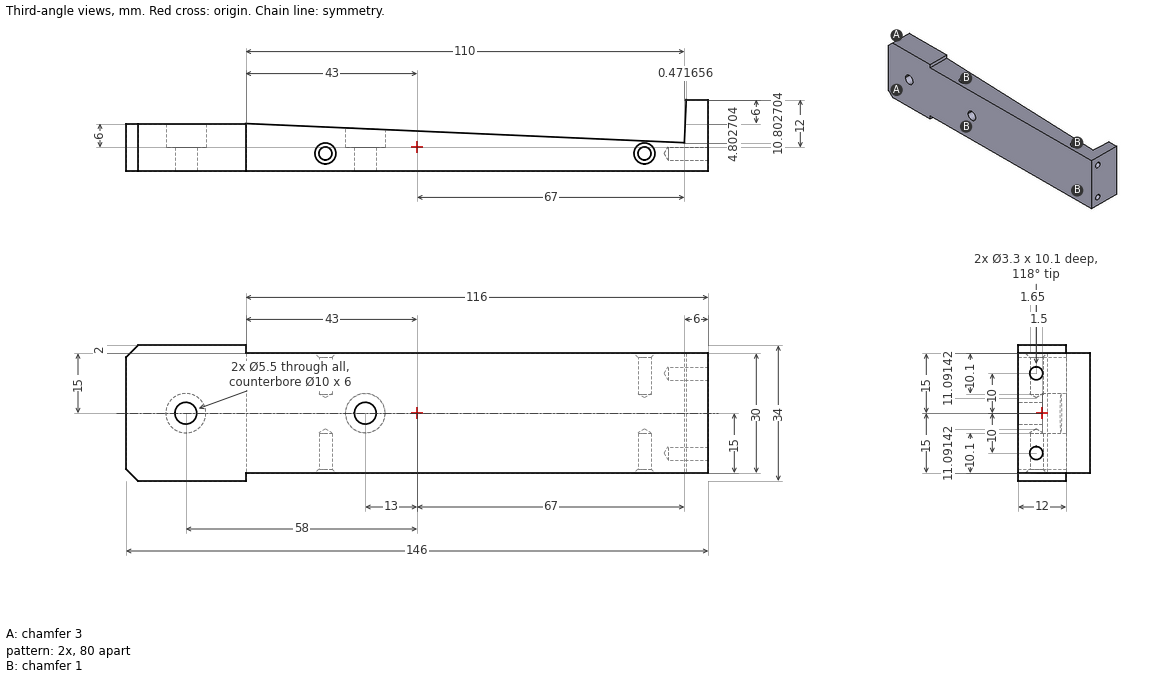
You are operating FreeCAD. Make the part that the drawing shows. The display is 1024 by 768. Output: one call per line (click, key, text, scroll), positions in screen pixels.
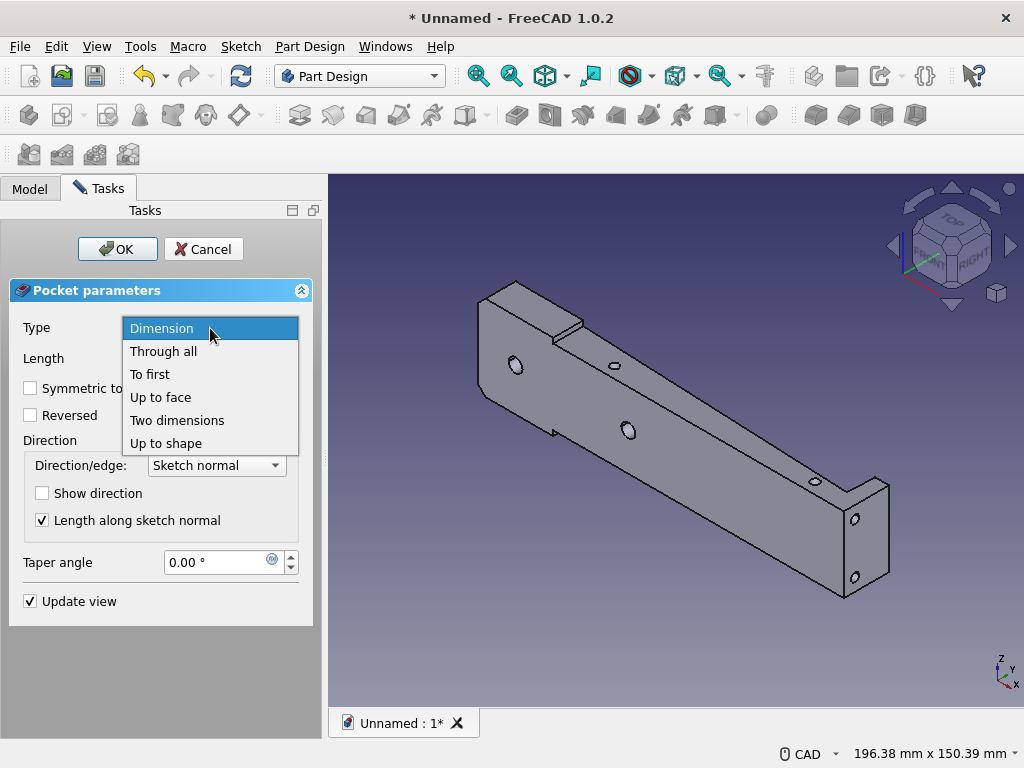
click(208, 352)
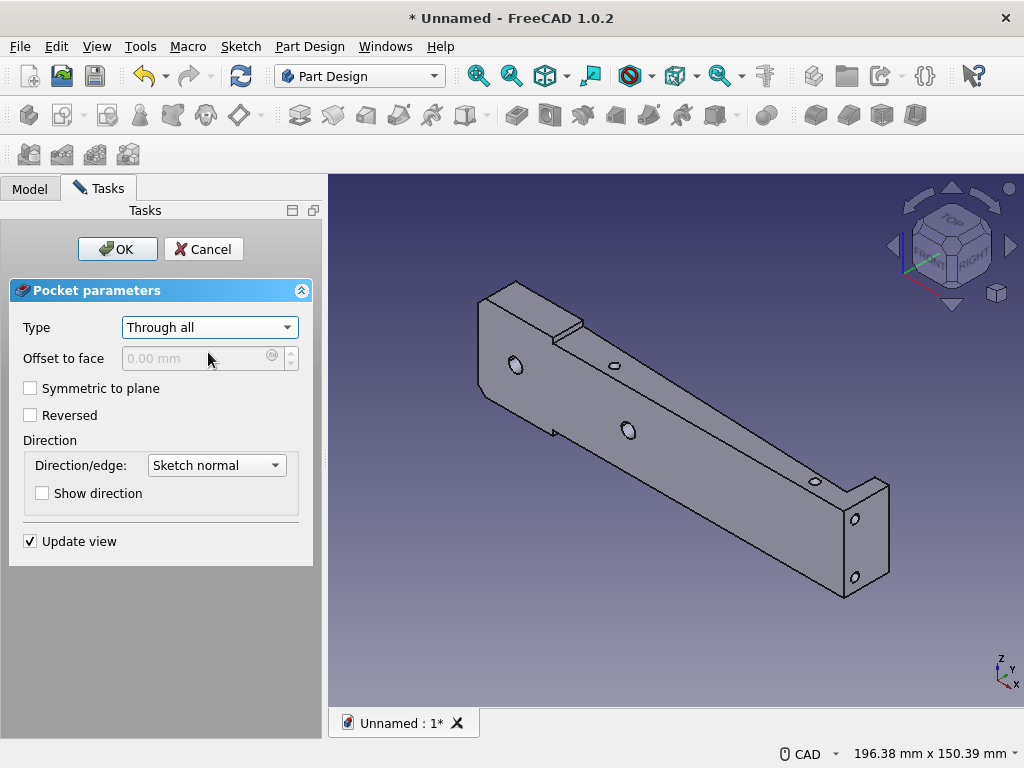
click(118, 249)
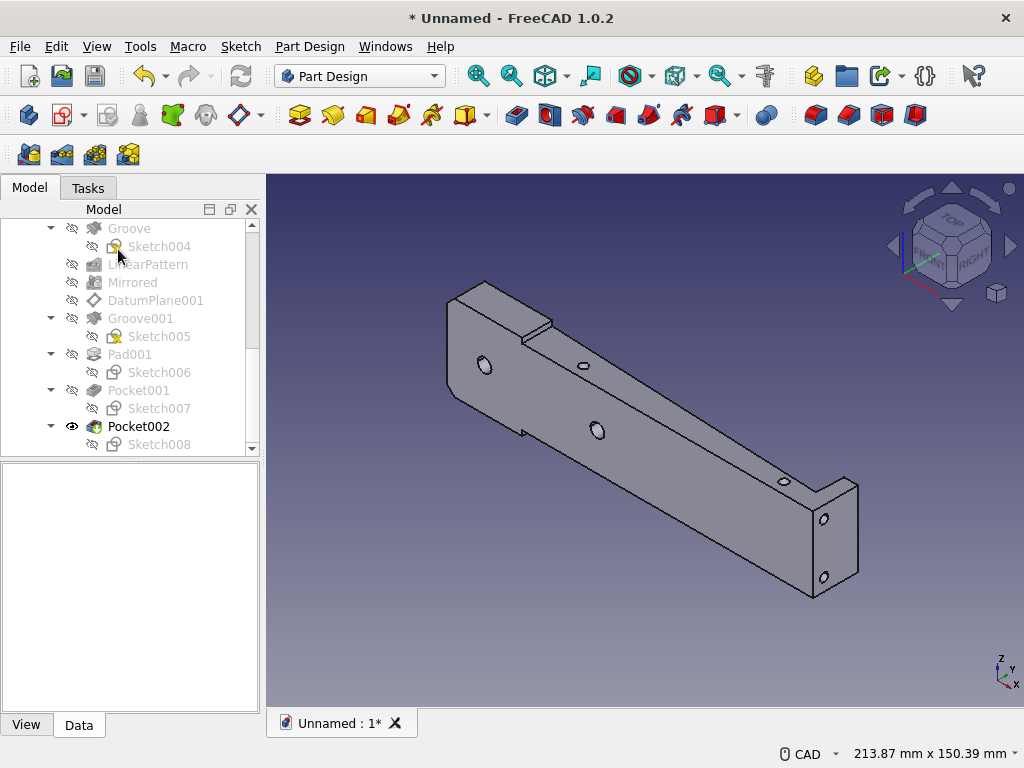
click(788, 478)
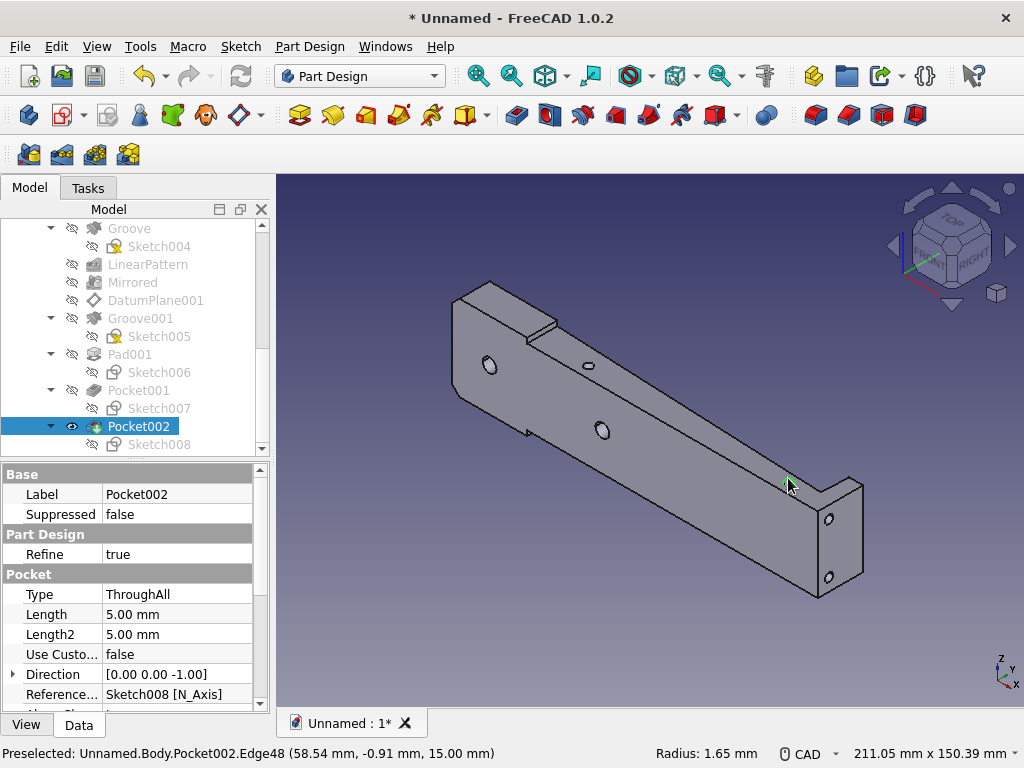
click(593, 363, ctrl)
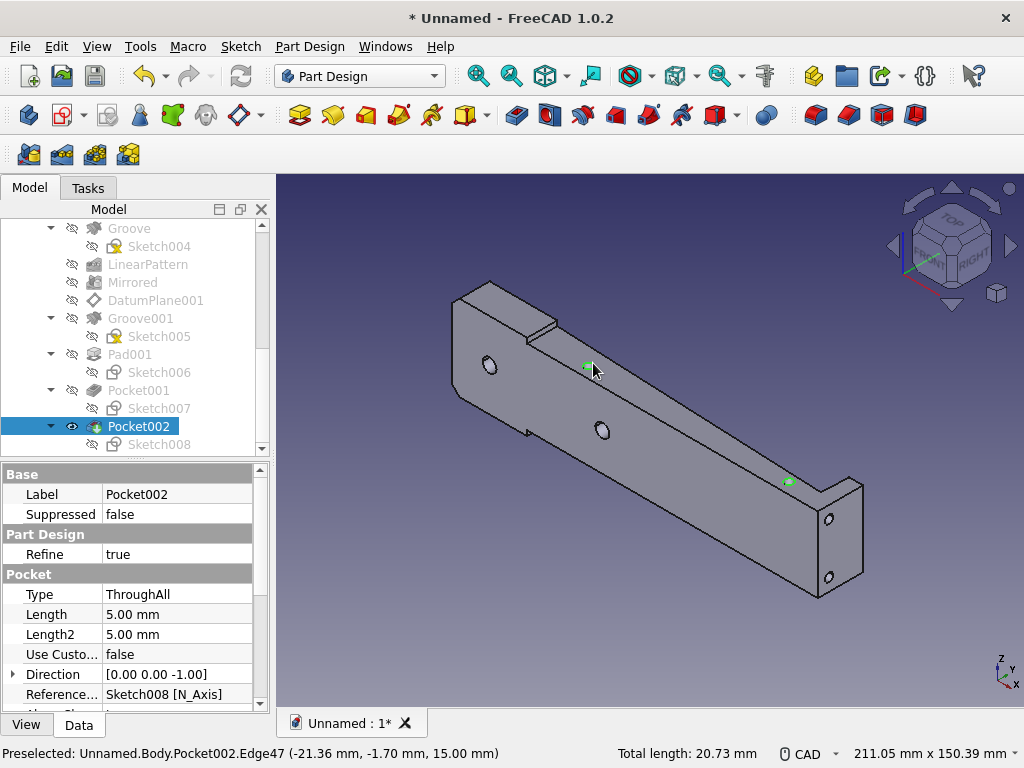
key(2)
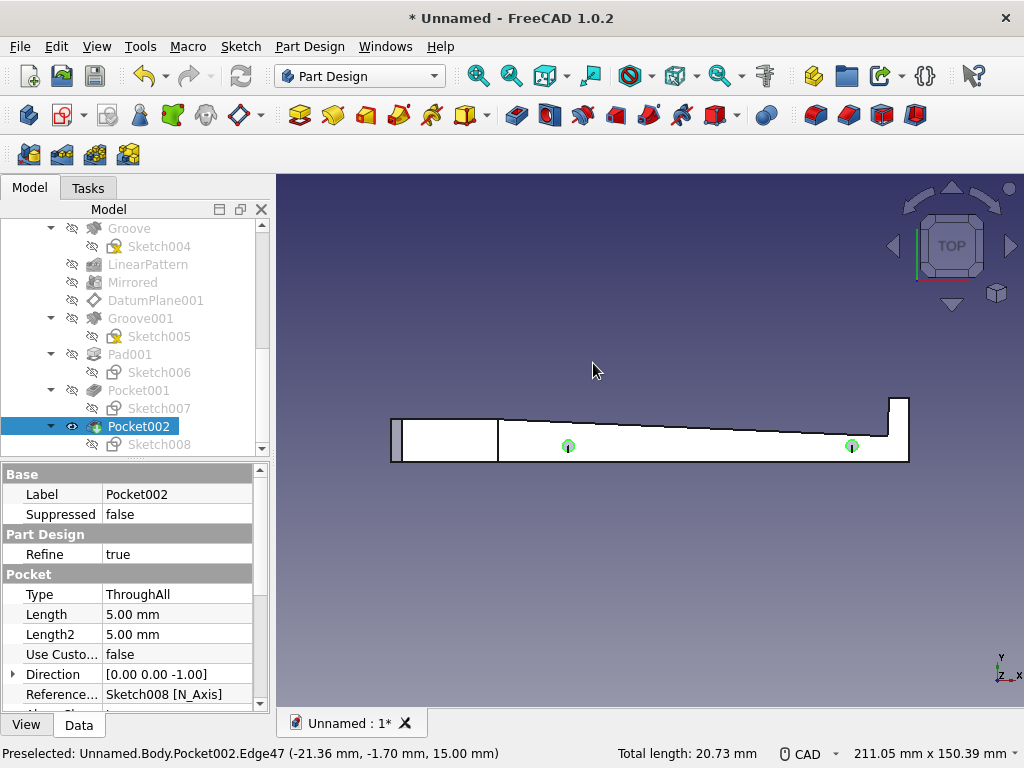
key(0)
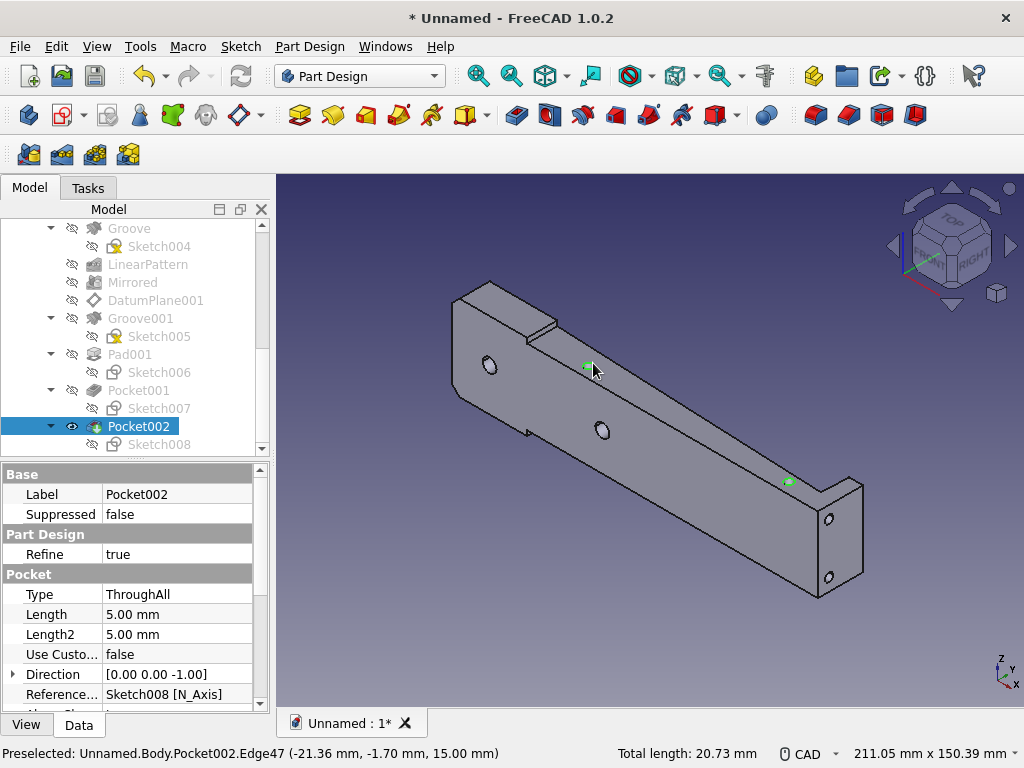
key(1)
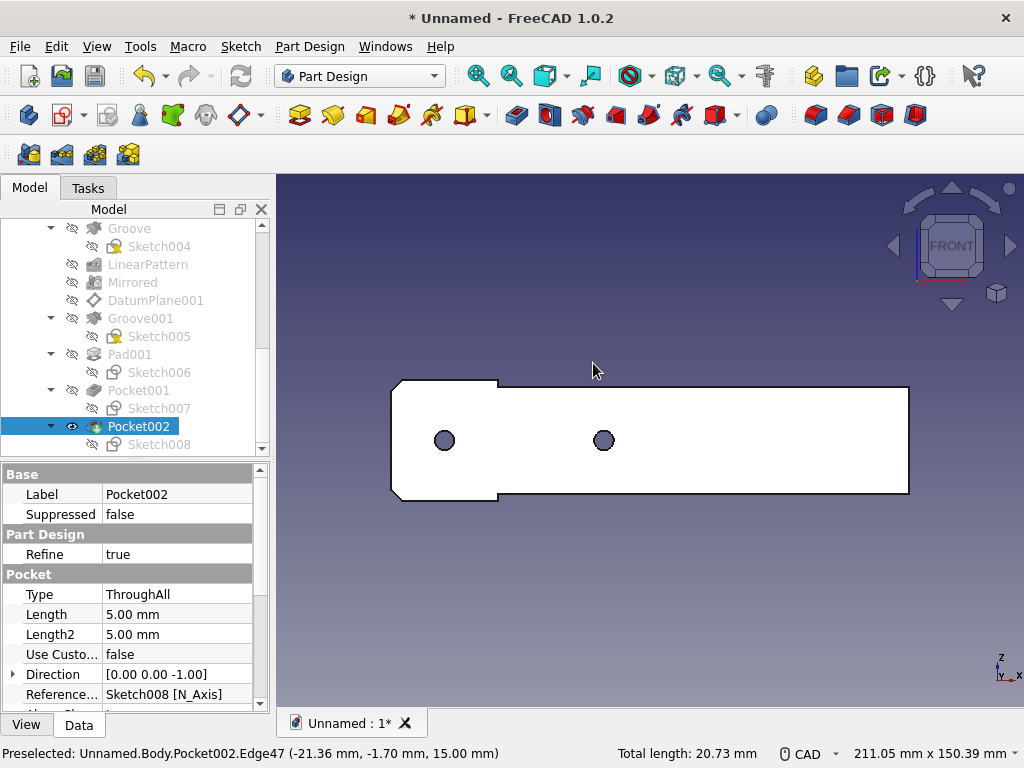
key(3)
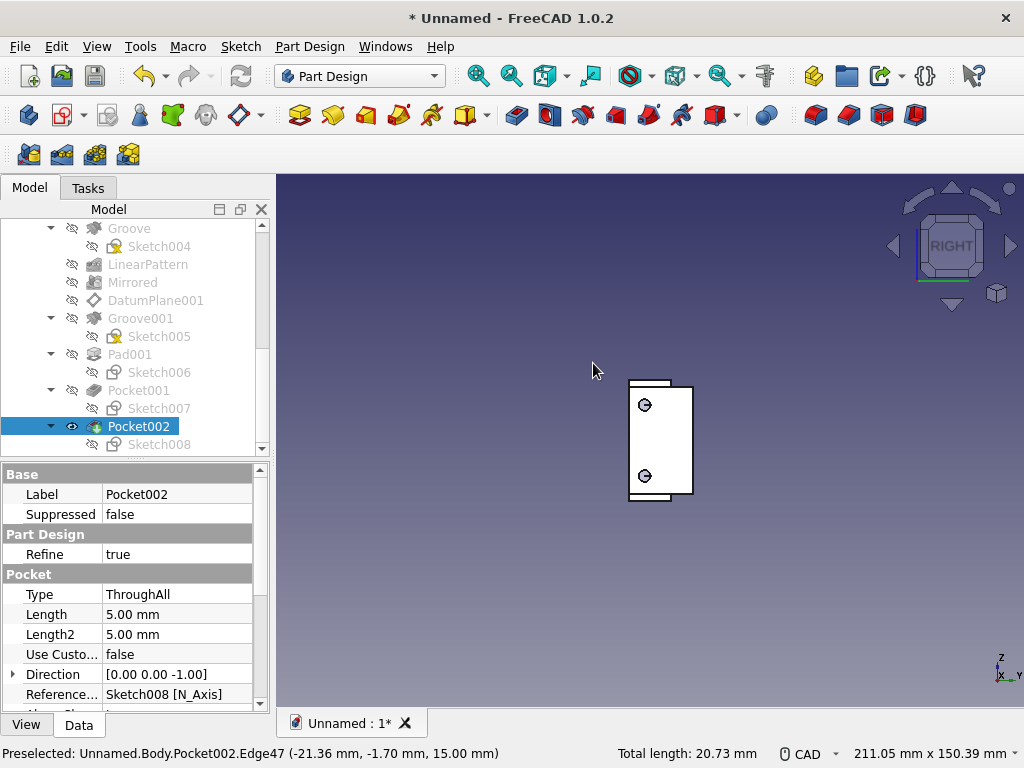
key(v)
key(f)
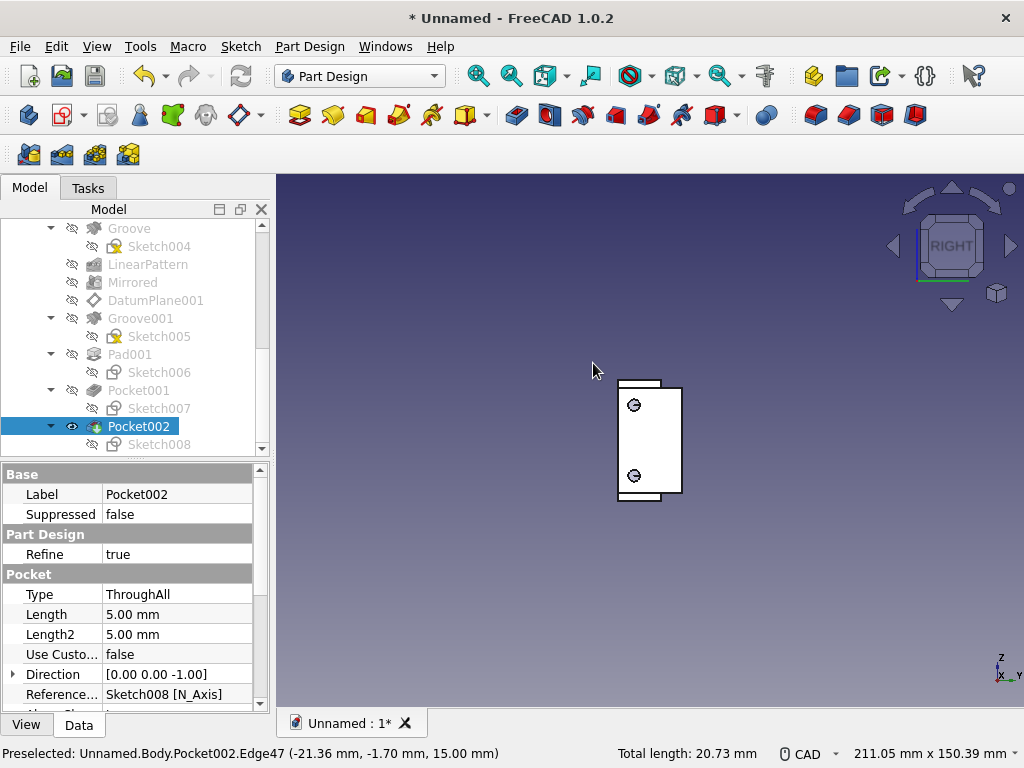
key(5)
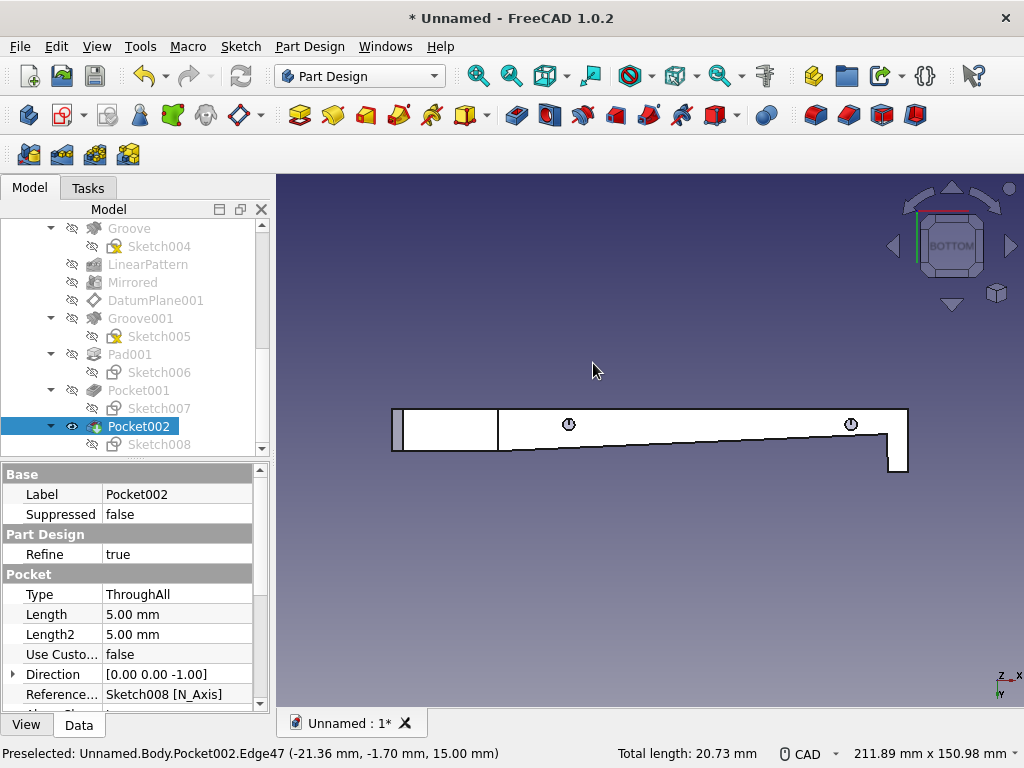
click(851, 429, ctrl)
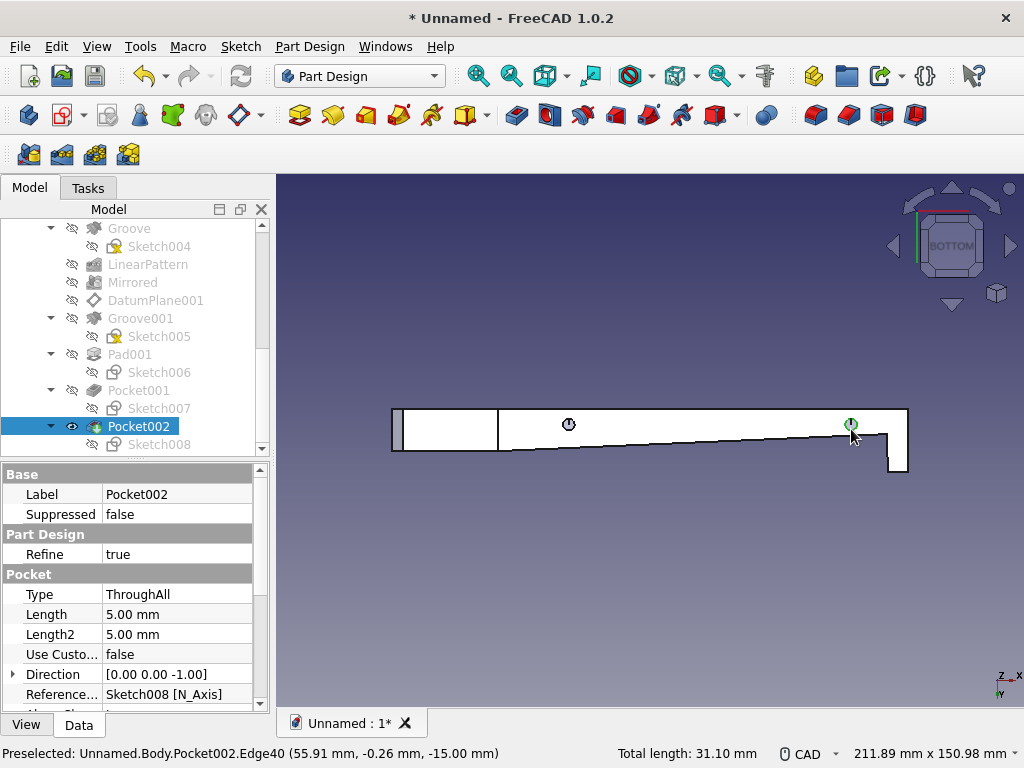
click(569, 429, ctrl)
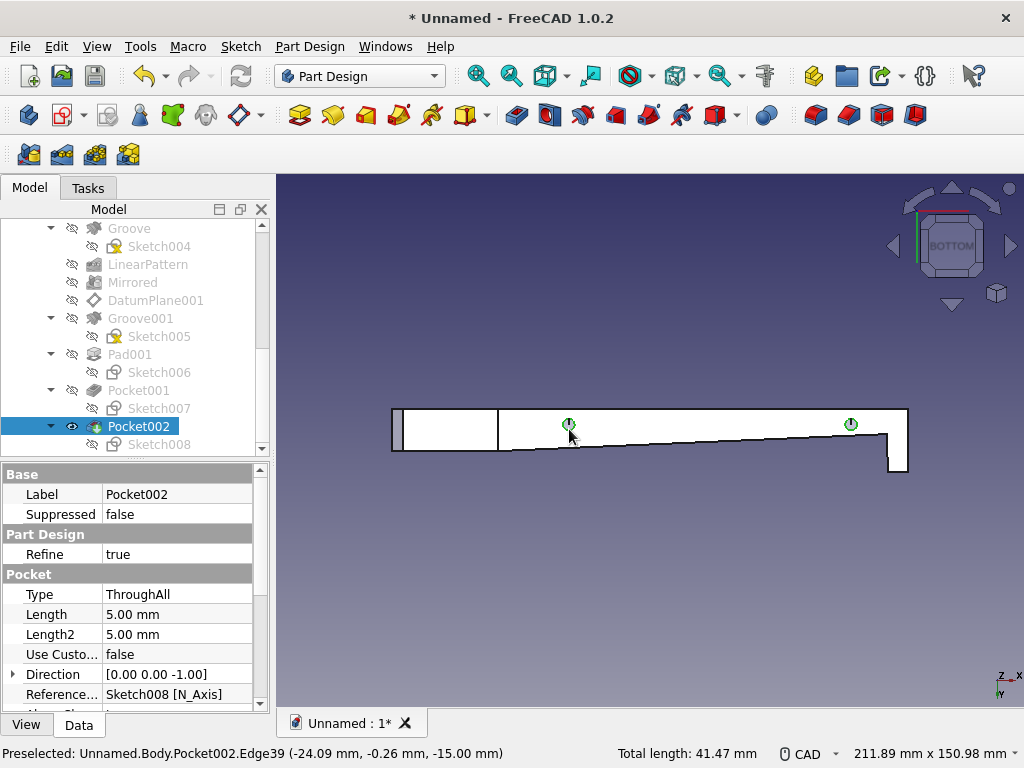
click(849, 116)